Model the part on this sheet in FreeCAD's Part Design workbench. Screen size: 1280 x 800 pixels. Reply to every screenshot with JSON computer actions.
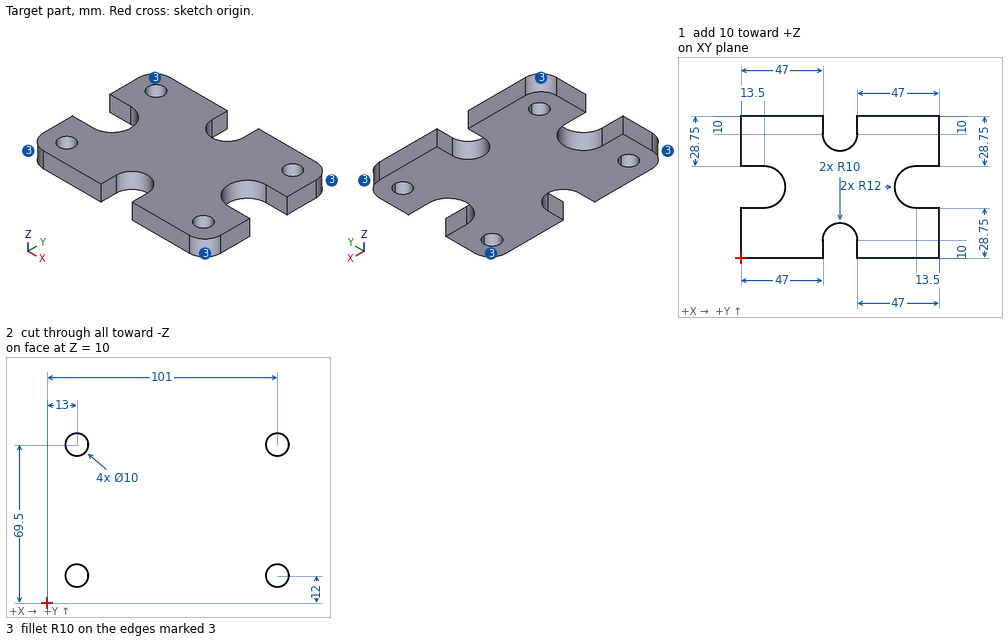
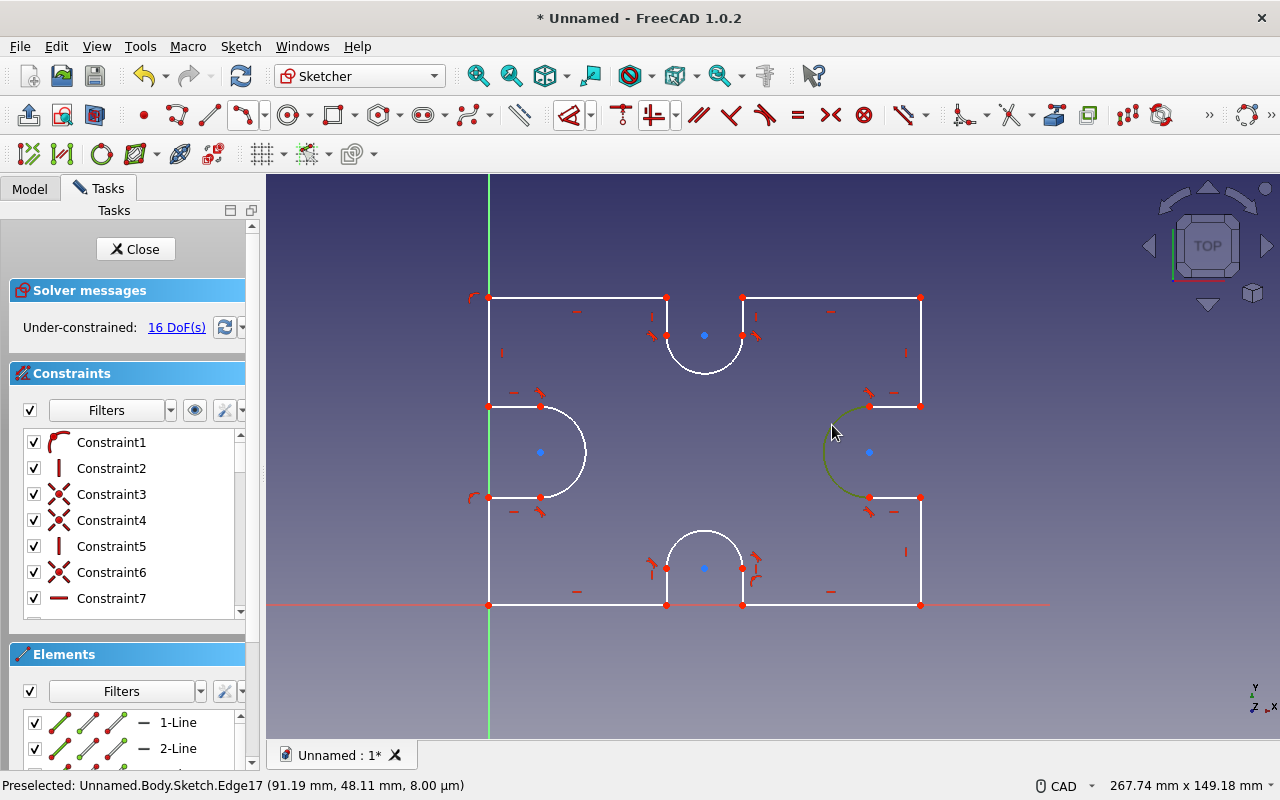
{"action": "left_click", "coordinate": [577, 479]}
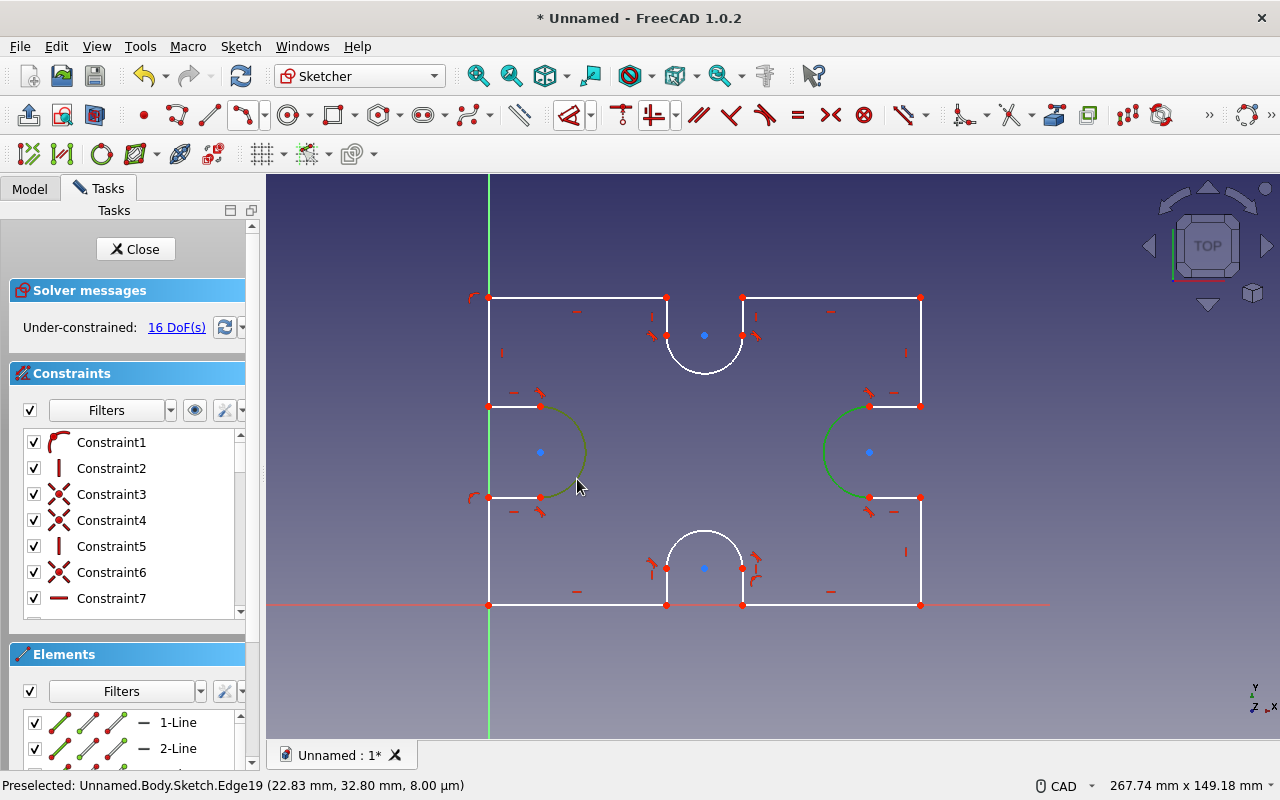
{"action": "left_click", "coordinate": [798, 116]}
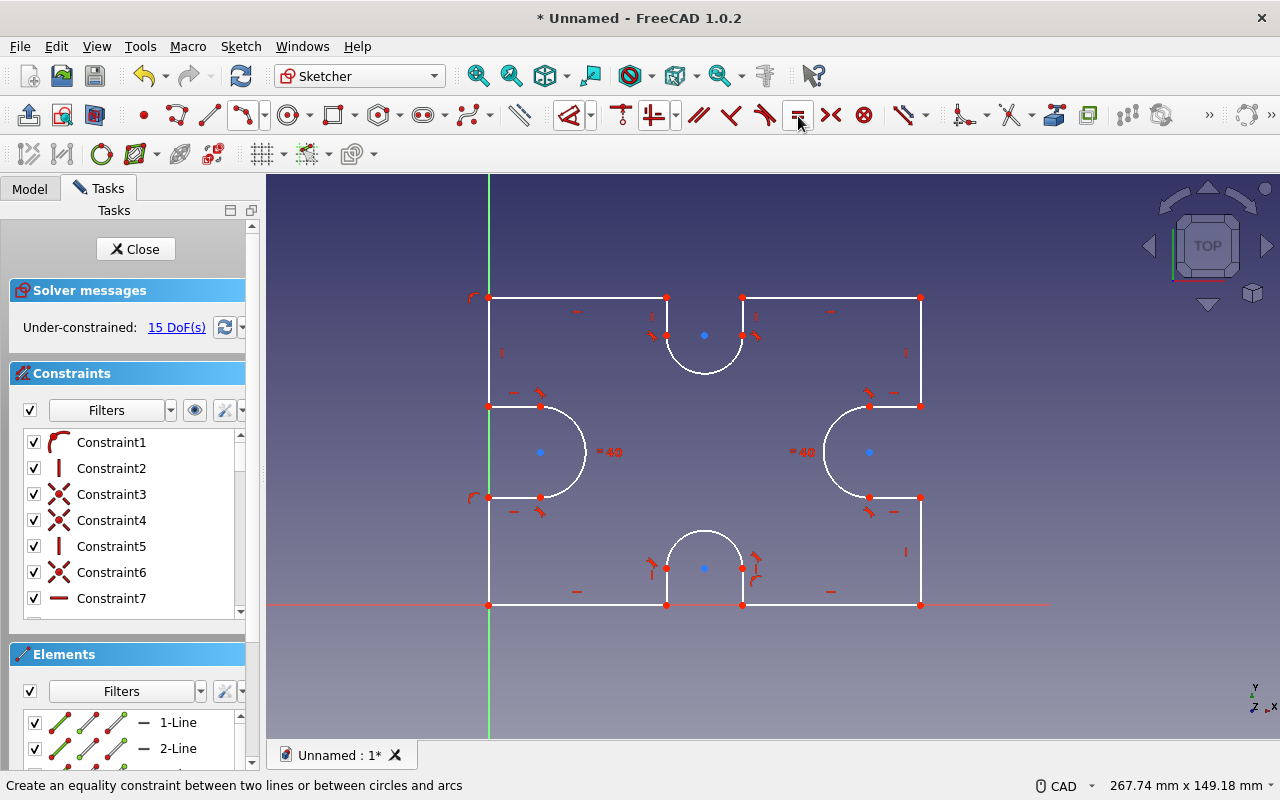
{"action": "left_click", "coordinate": [682, 366]}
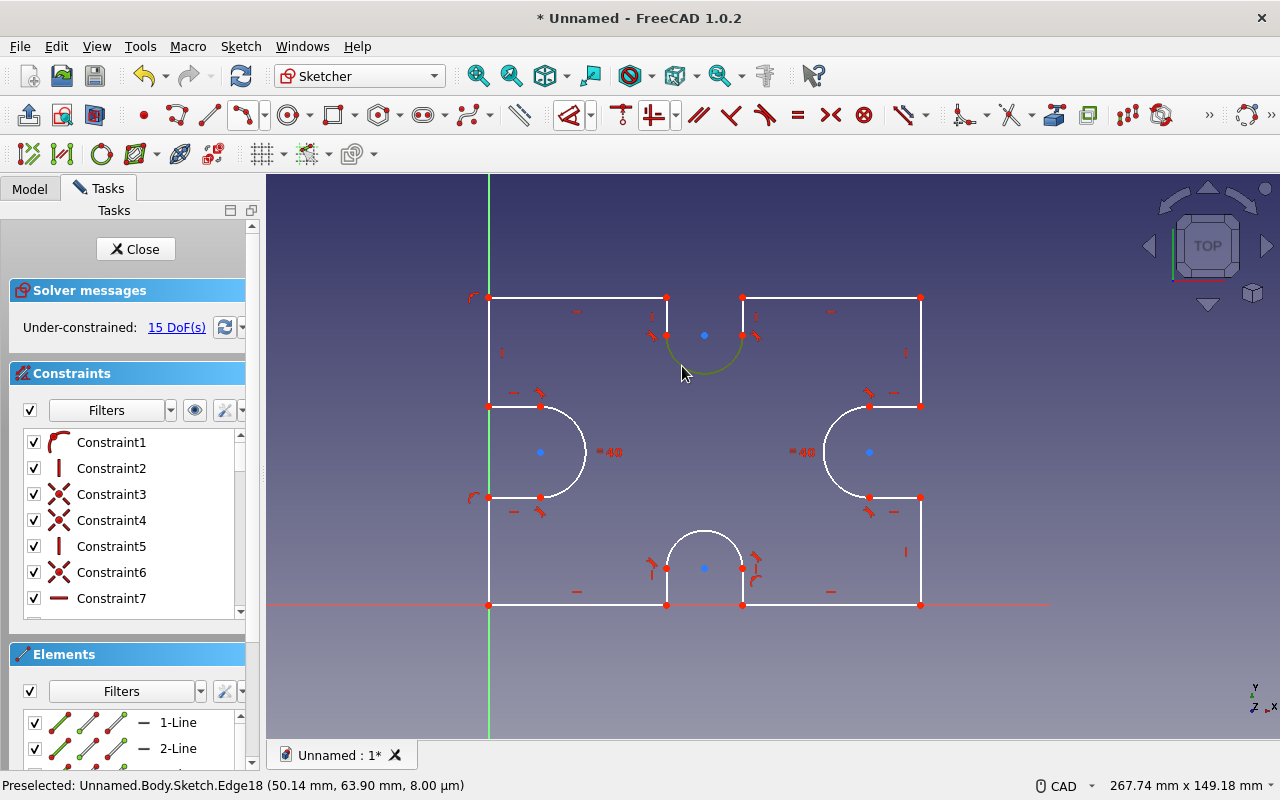
{"action": "left_click", "coordinate": [727, 538]}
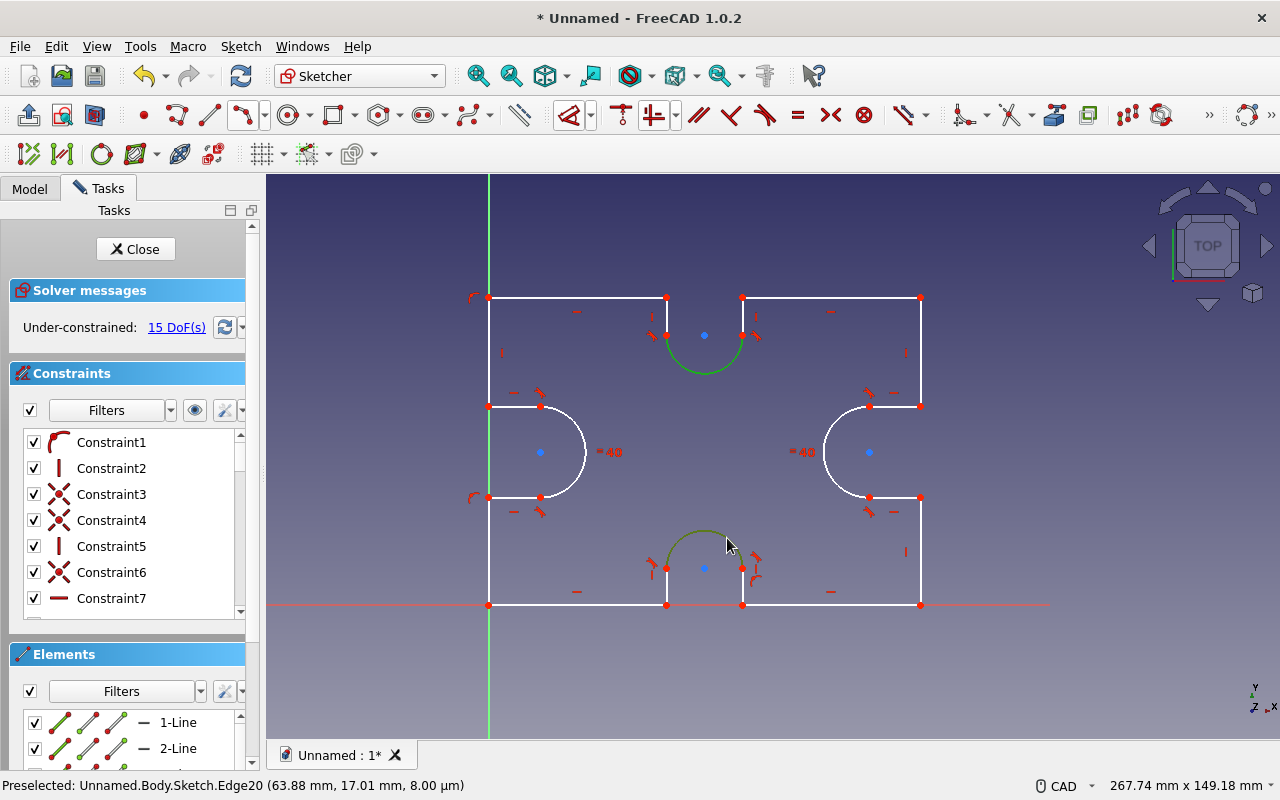
{"action": "left_click", "coordinate": [798, 116]}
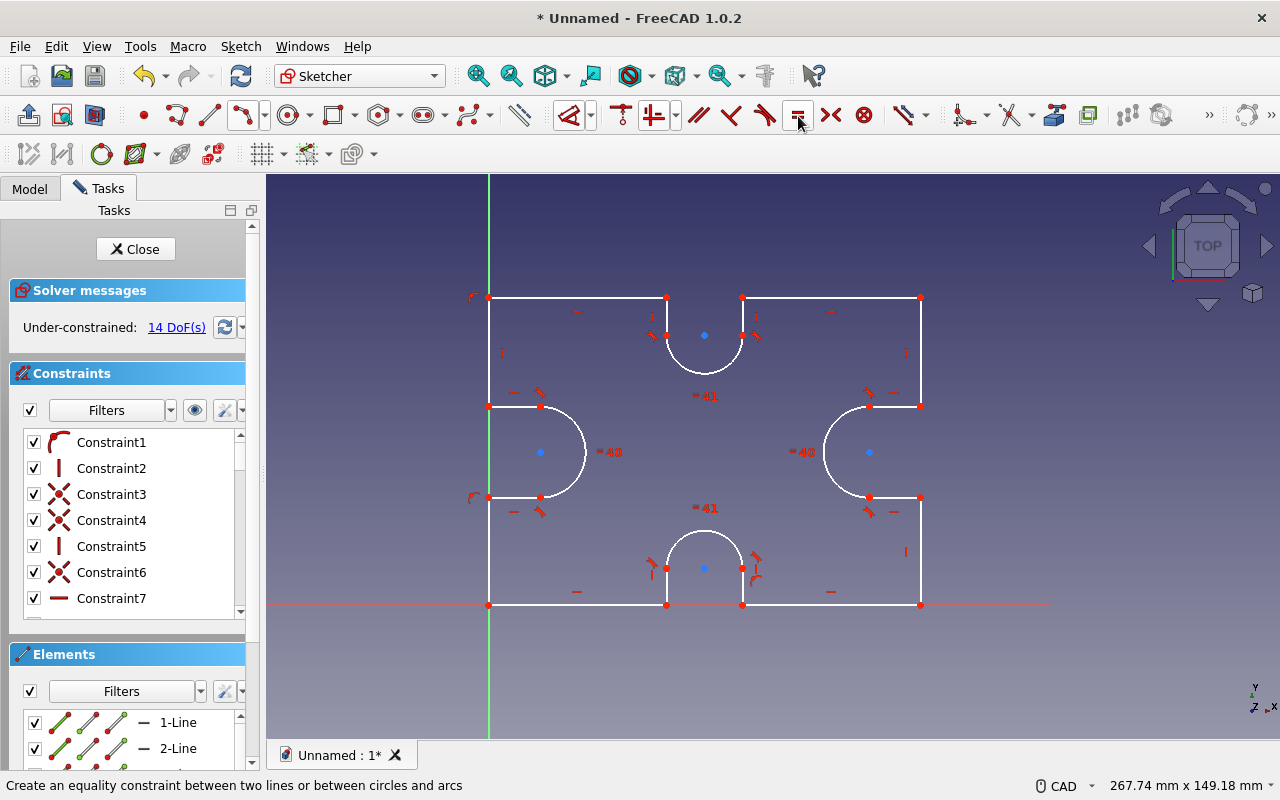
{"action": "left_click", "coordinate": [832, 425]}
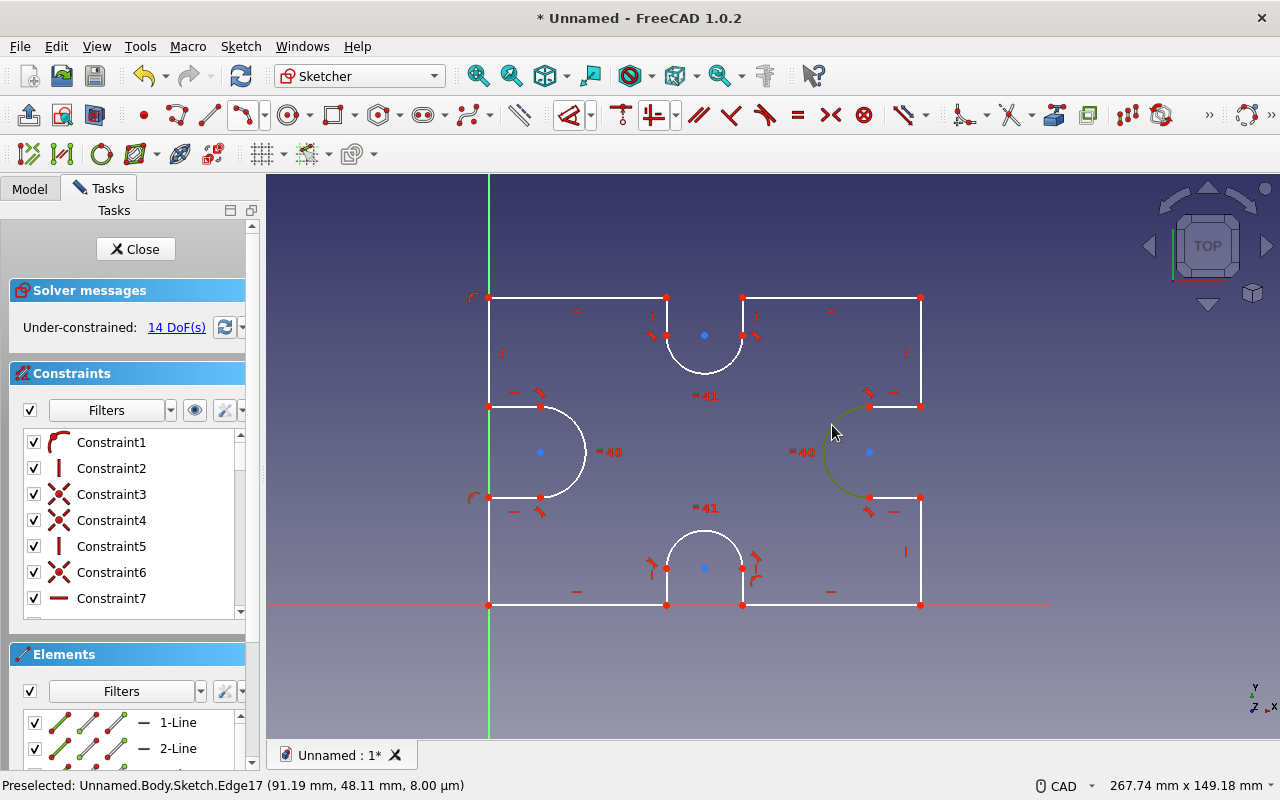
{"action": "left_click", "coordinate": [590, 116]}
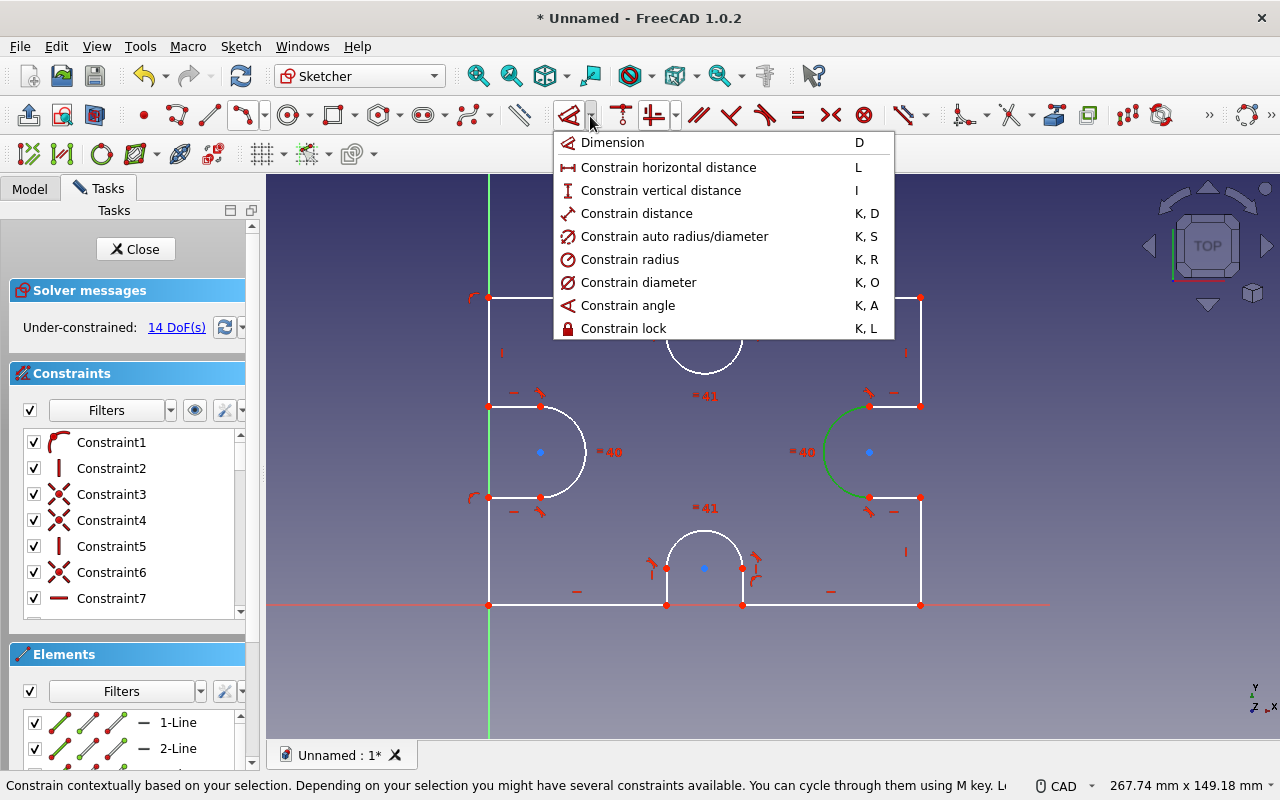
{"action": "left_click", "coordinate": [724, 260]}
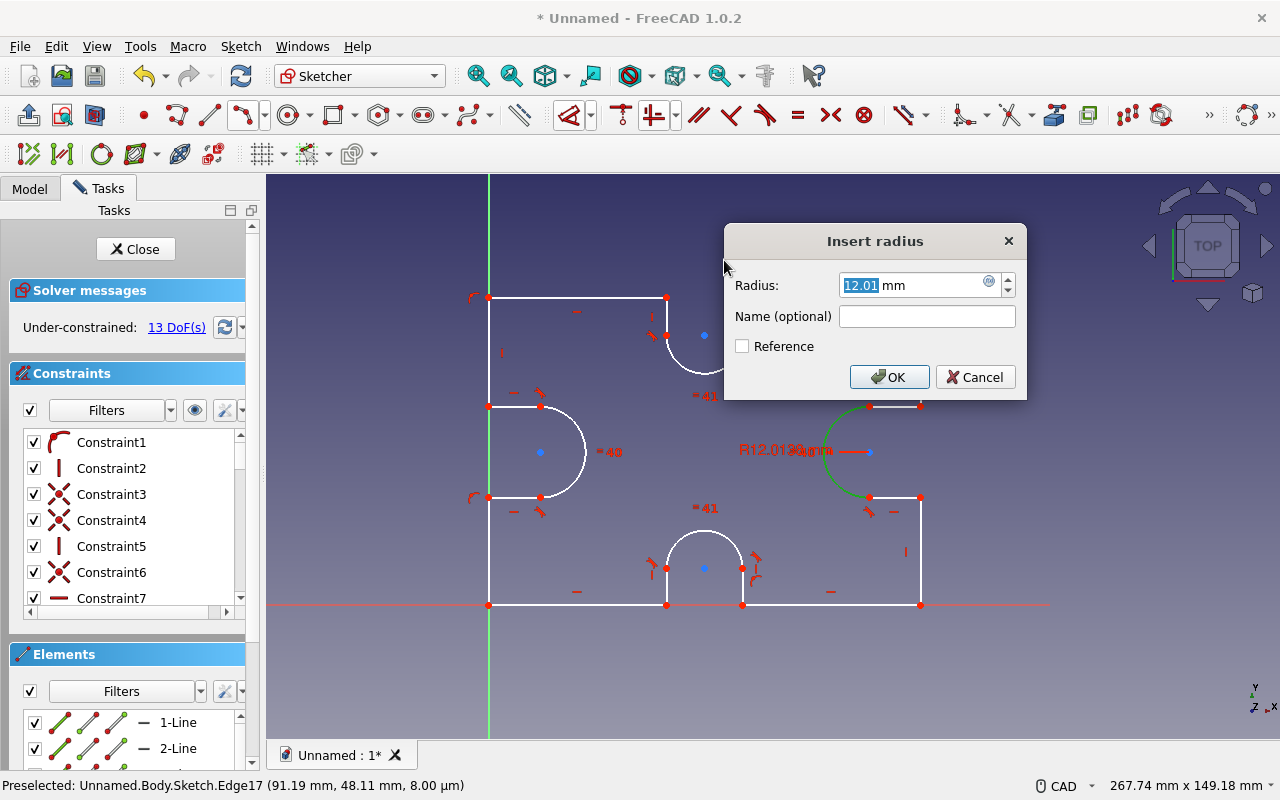
{"action": "type", "text": "12"}
{"action": "key", "text": "Return"}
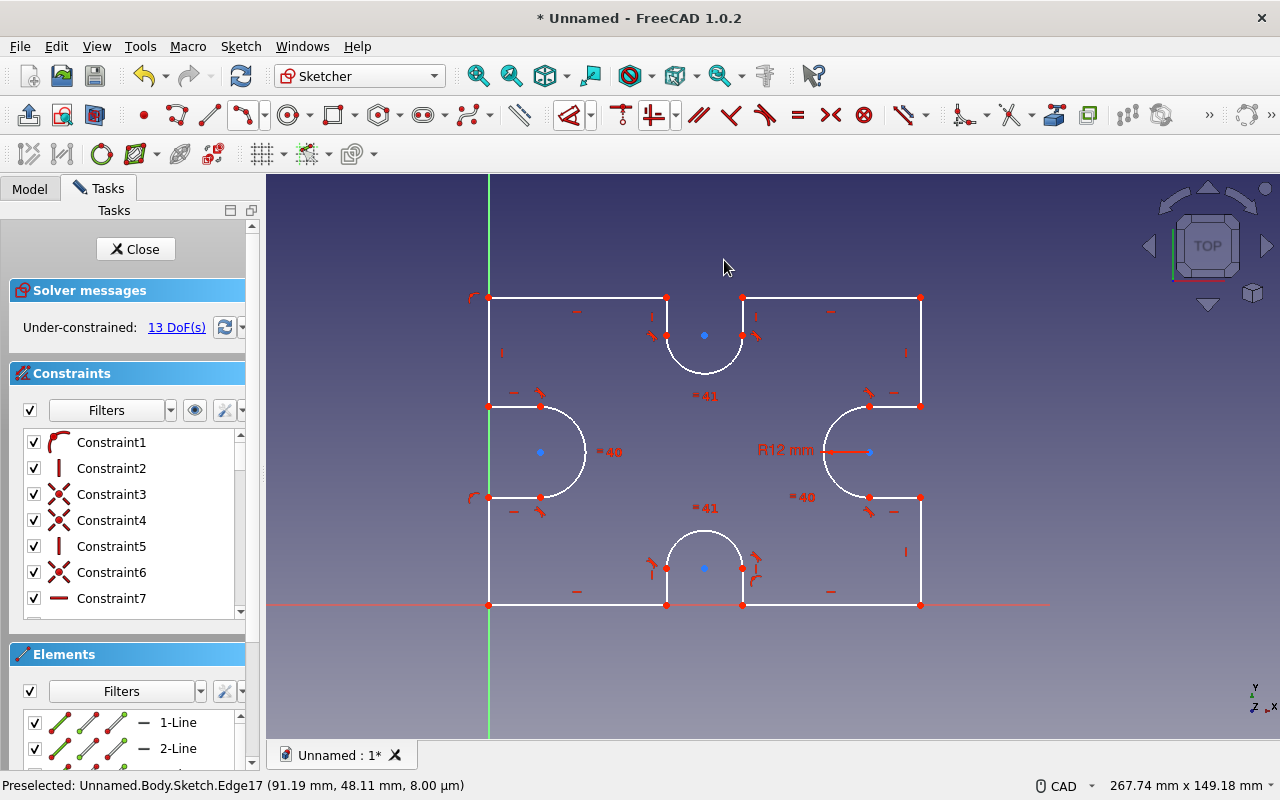
{"action": "left_click", "coordinate": [682, 366]}